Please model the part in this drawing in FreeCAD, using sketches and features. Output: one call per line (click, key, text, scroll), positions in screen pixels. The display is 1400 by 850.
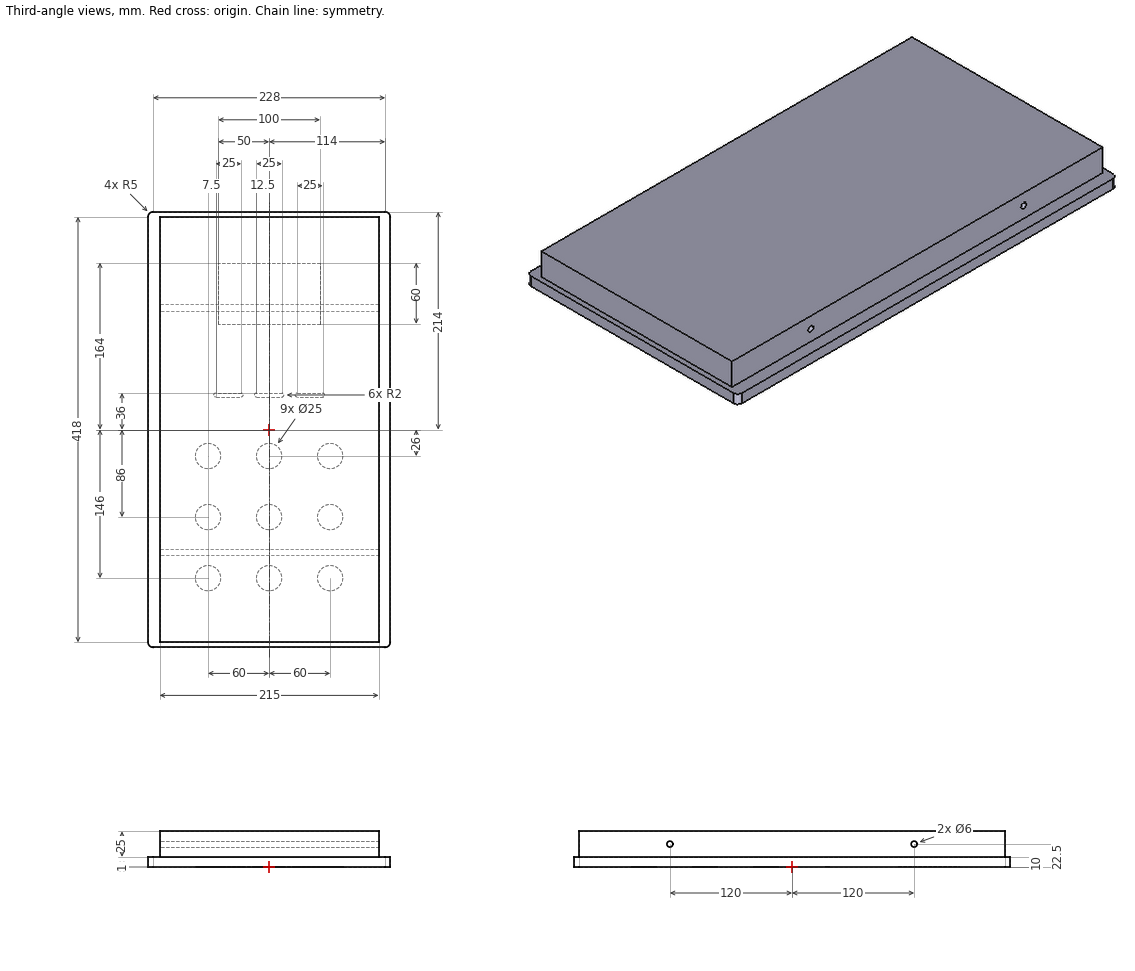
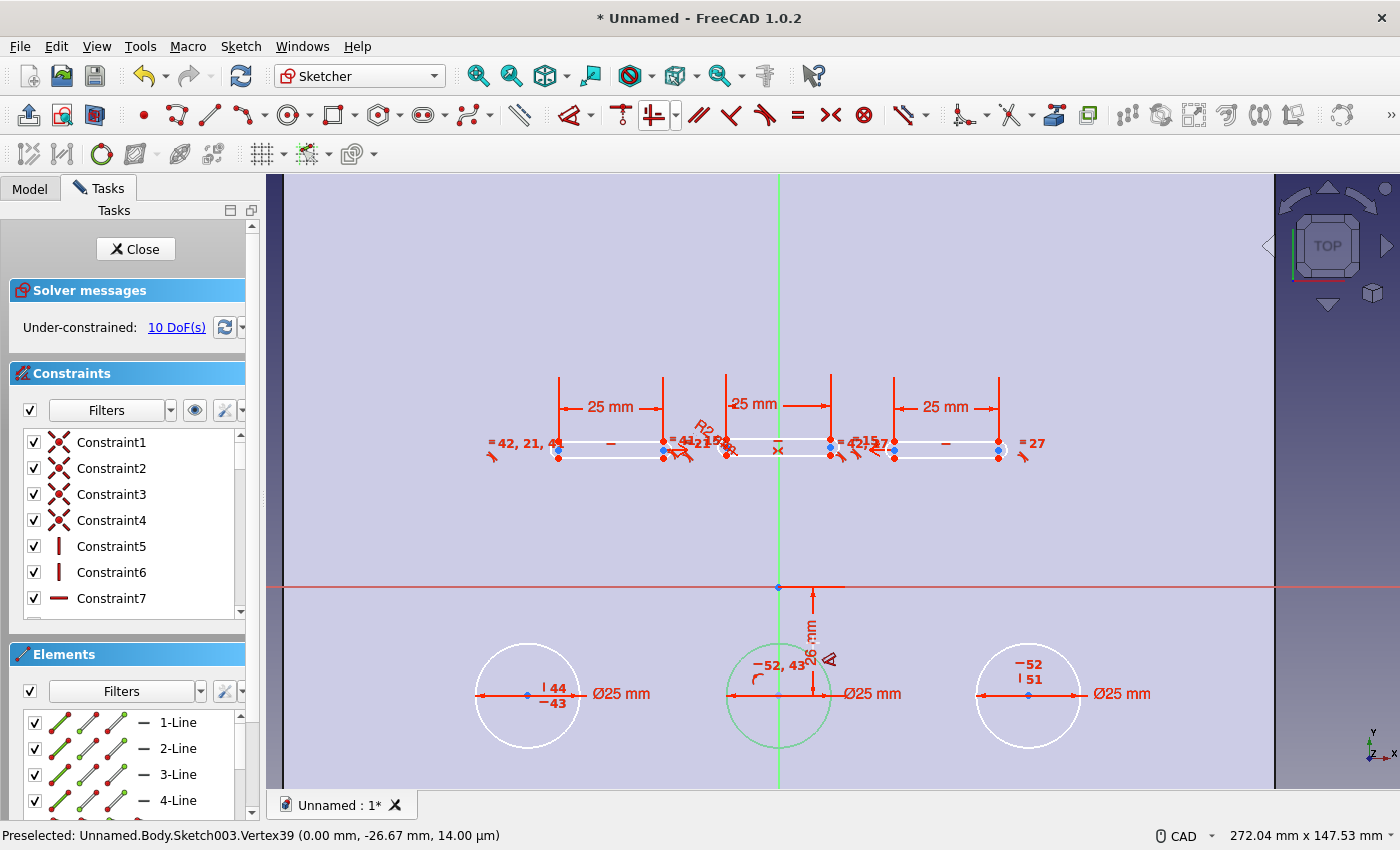
click(528, 696)
click(653, 730)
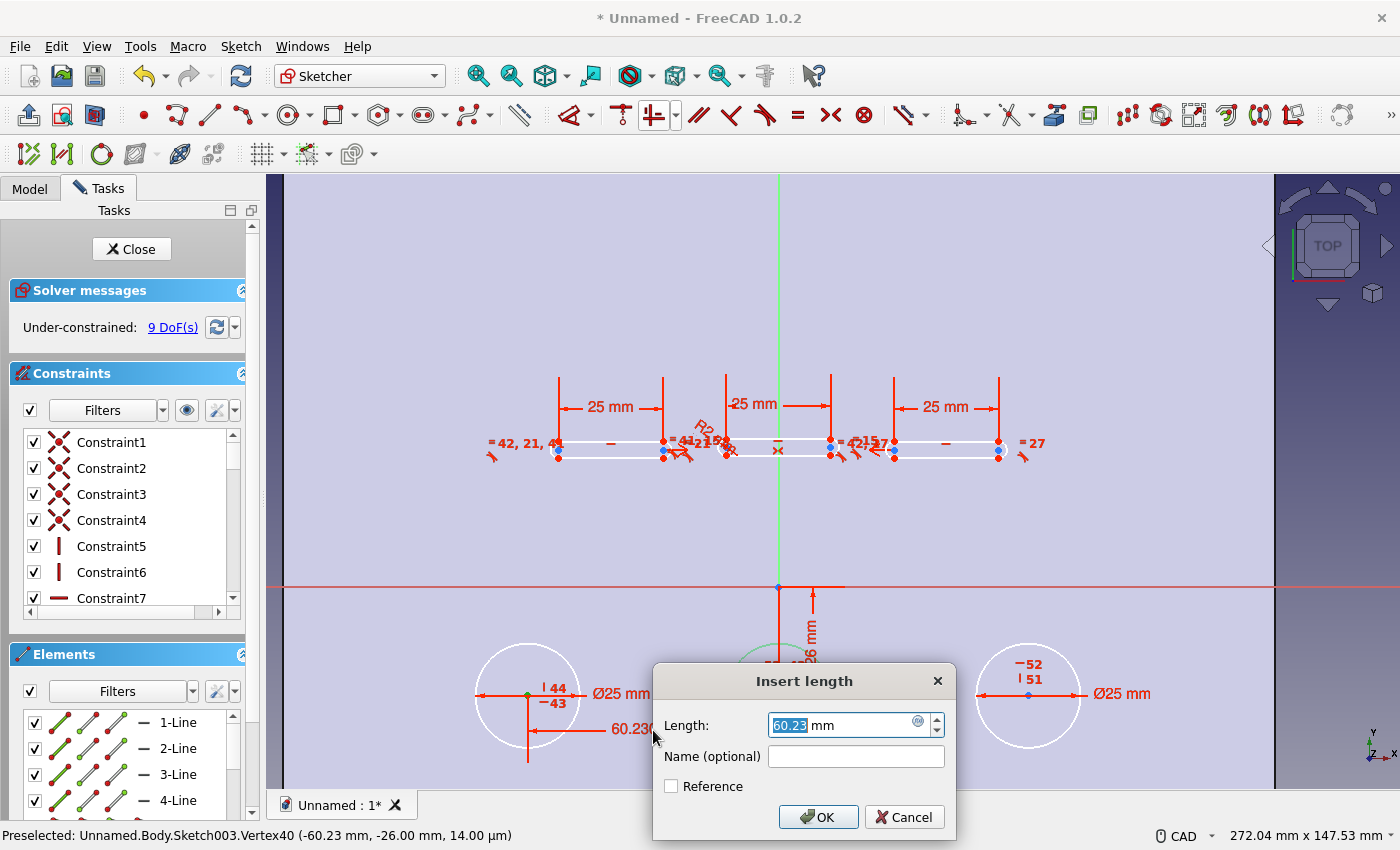
text(60)
key(Return)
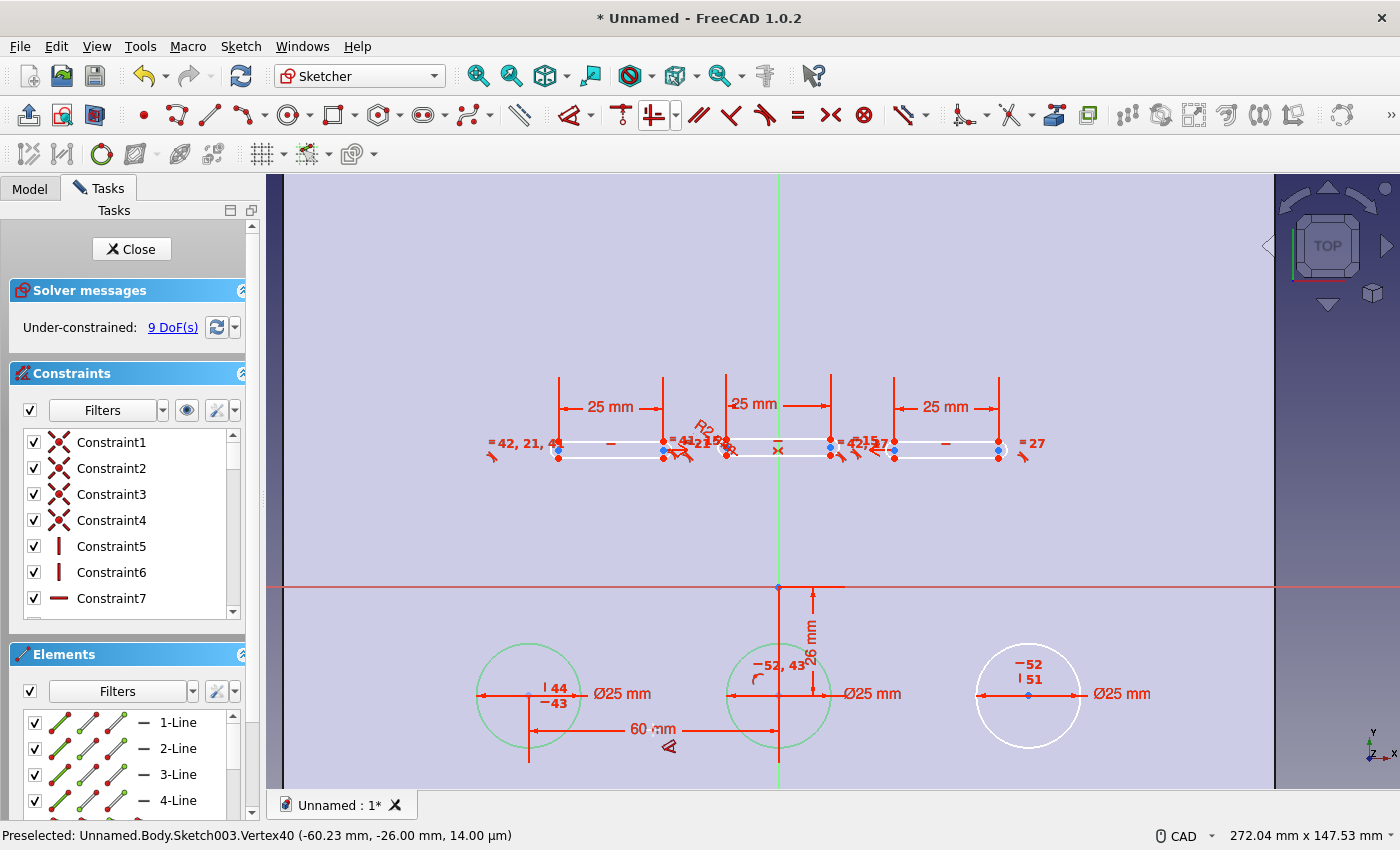
scroll(758, 441, down, 6)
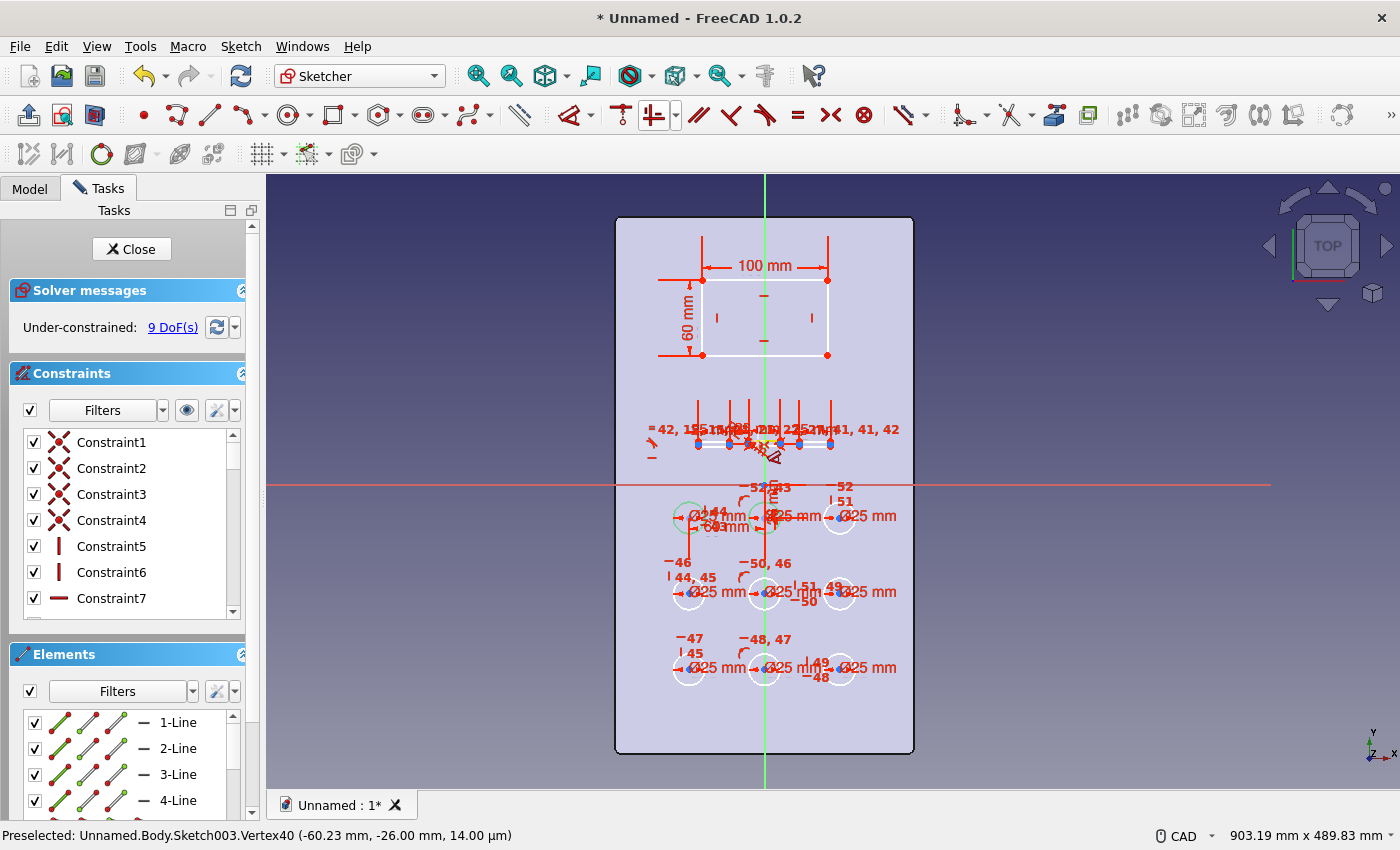
click(689, 594)
click(655, 540)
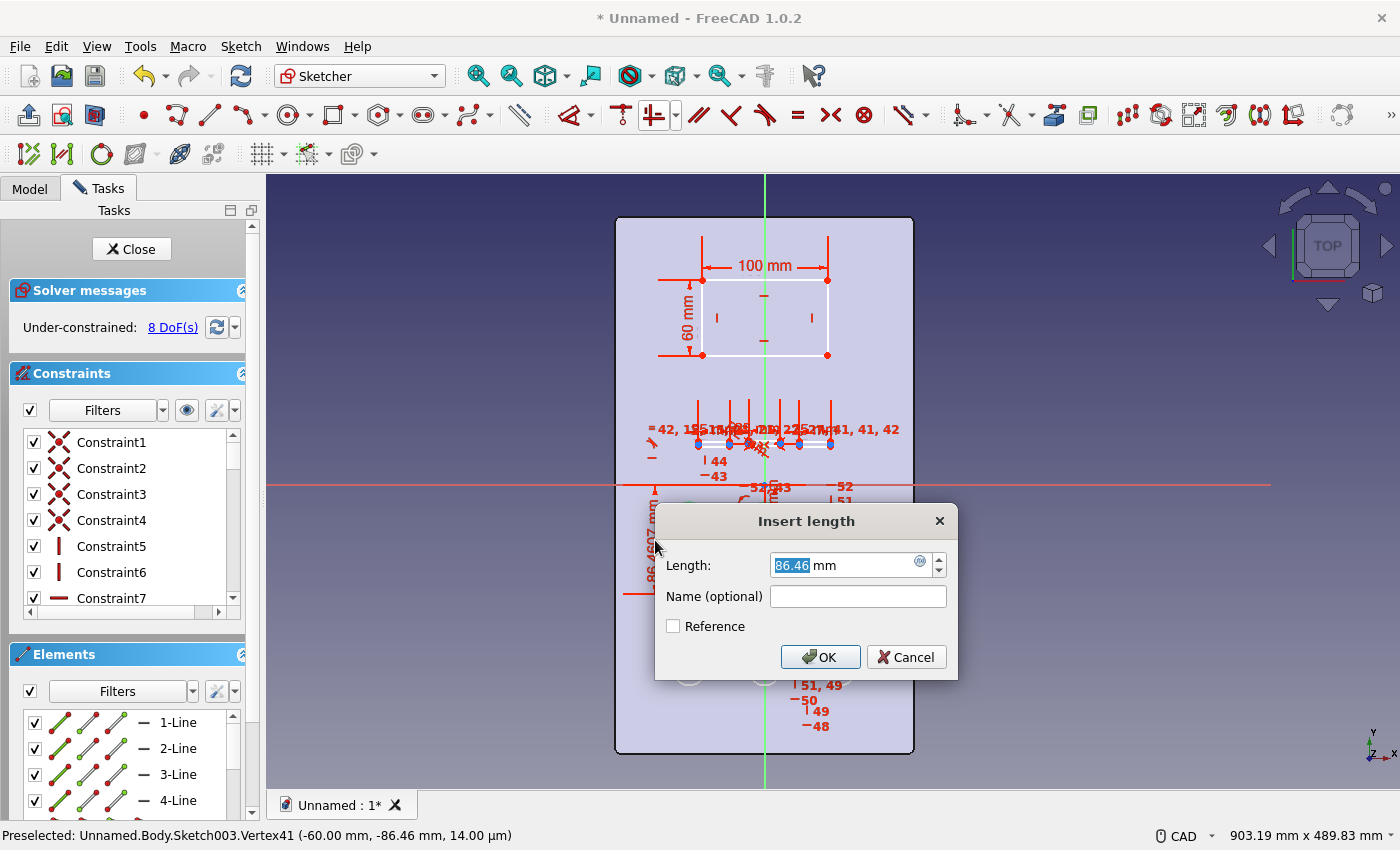
text(86)
key(Return)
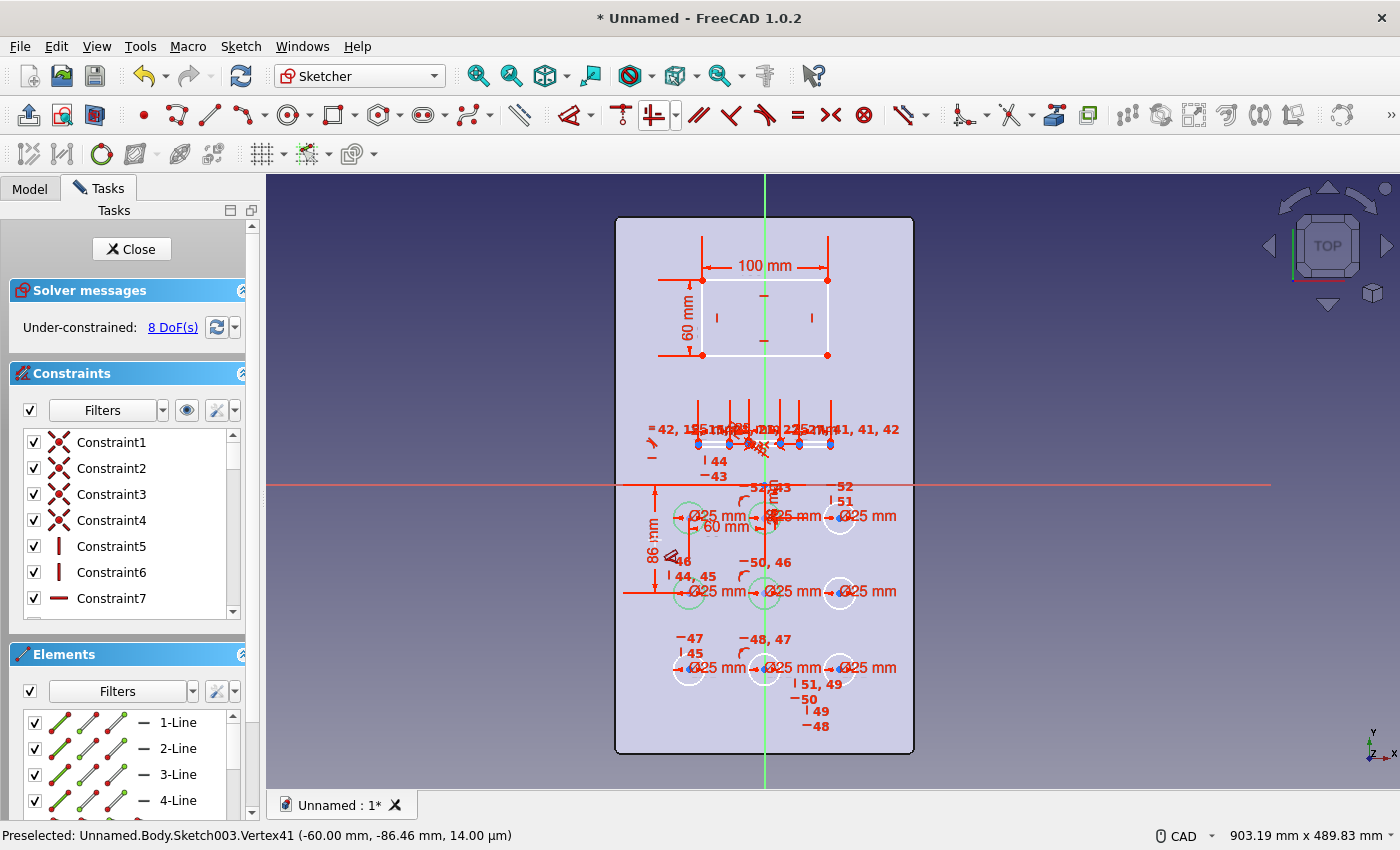
click(840, 670)
click(802, 704)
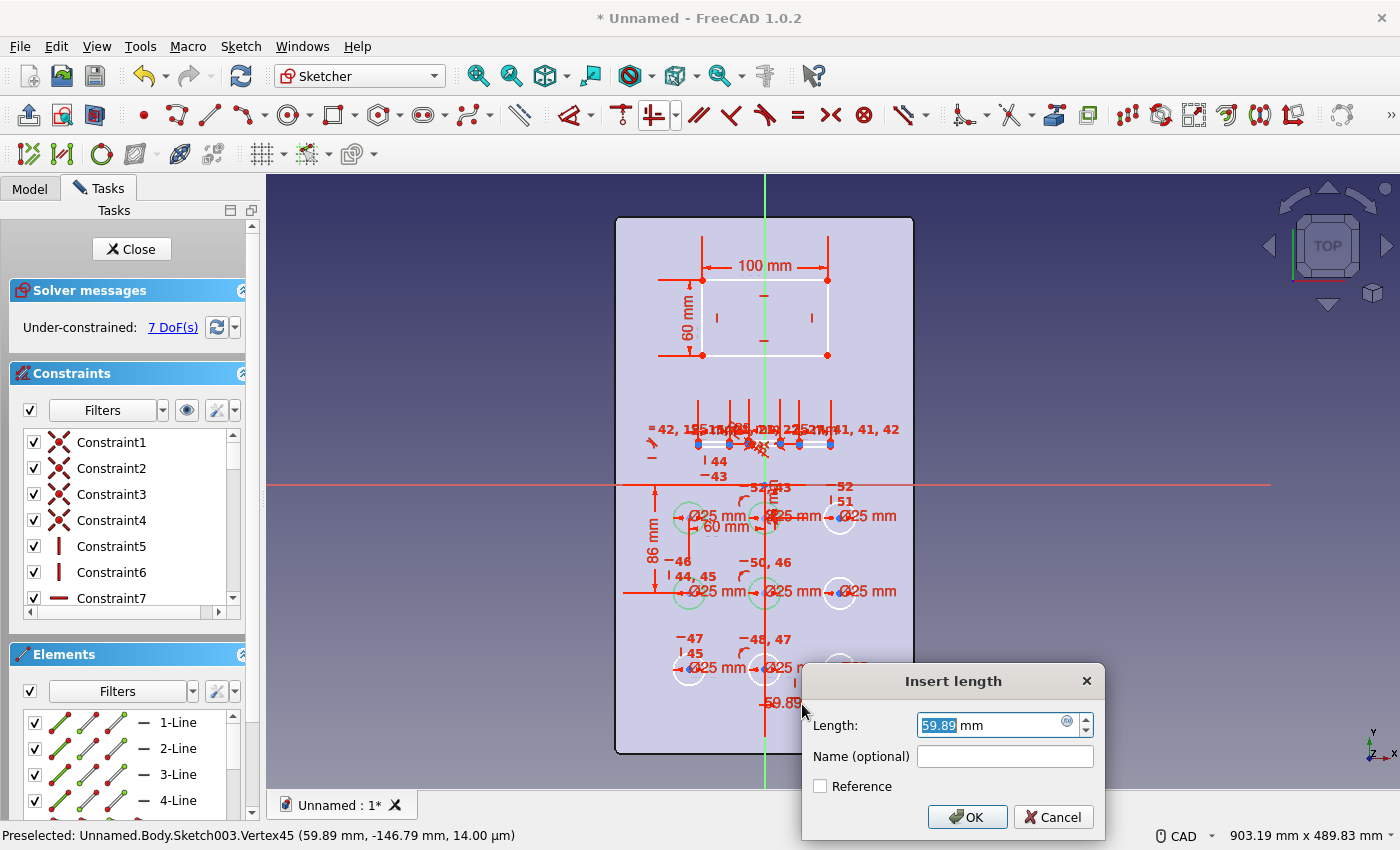
text(60)
key(Return)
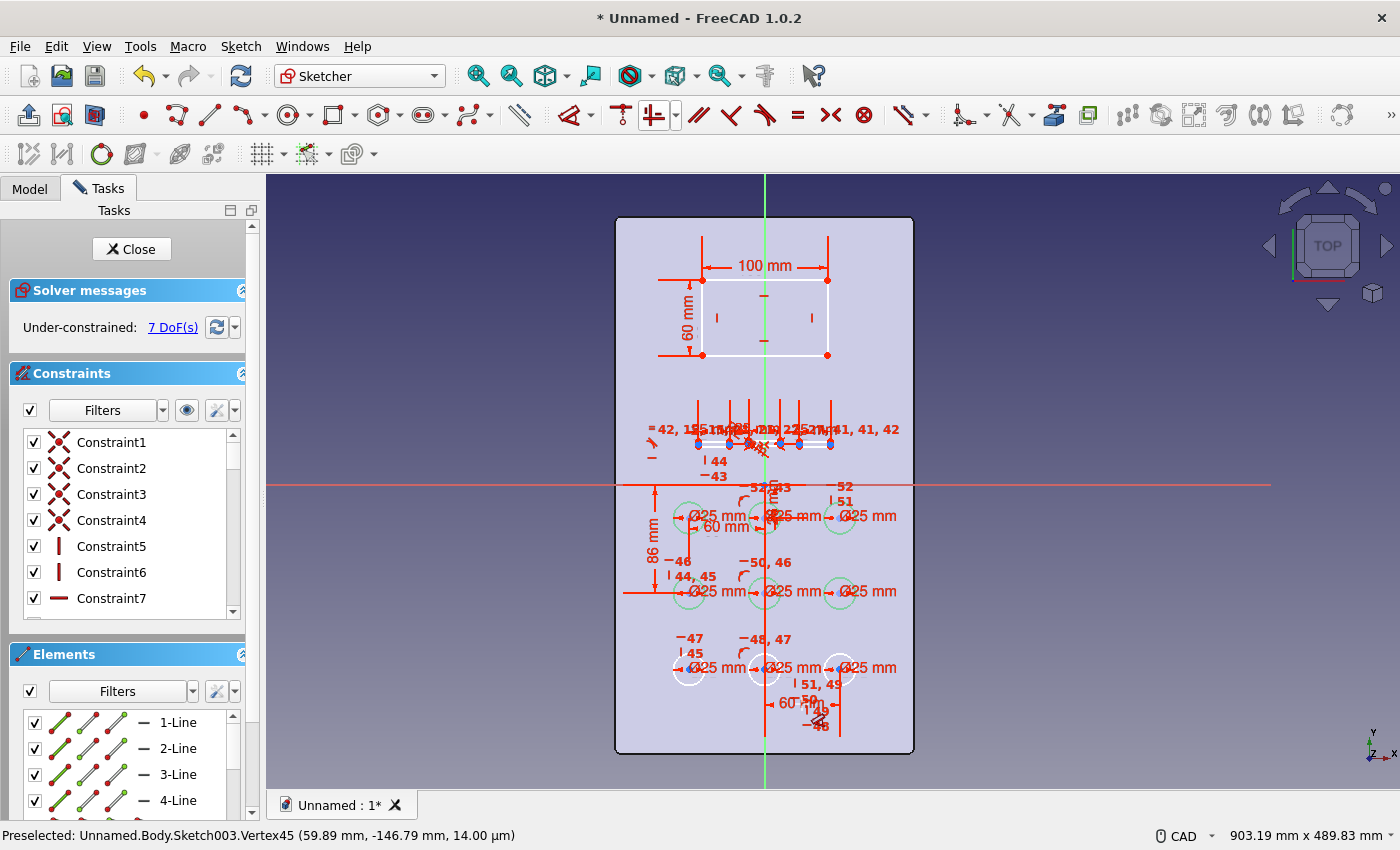
click(702, 280)
click(733, 246)